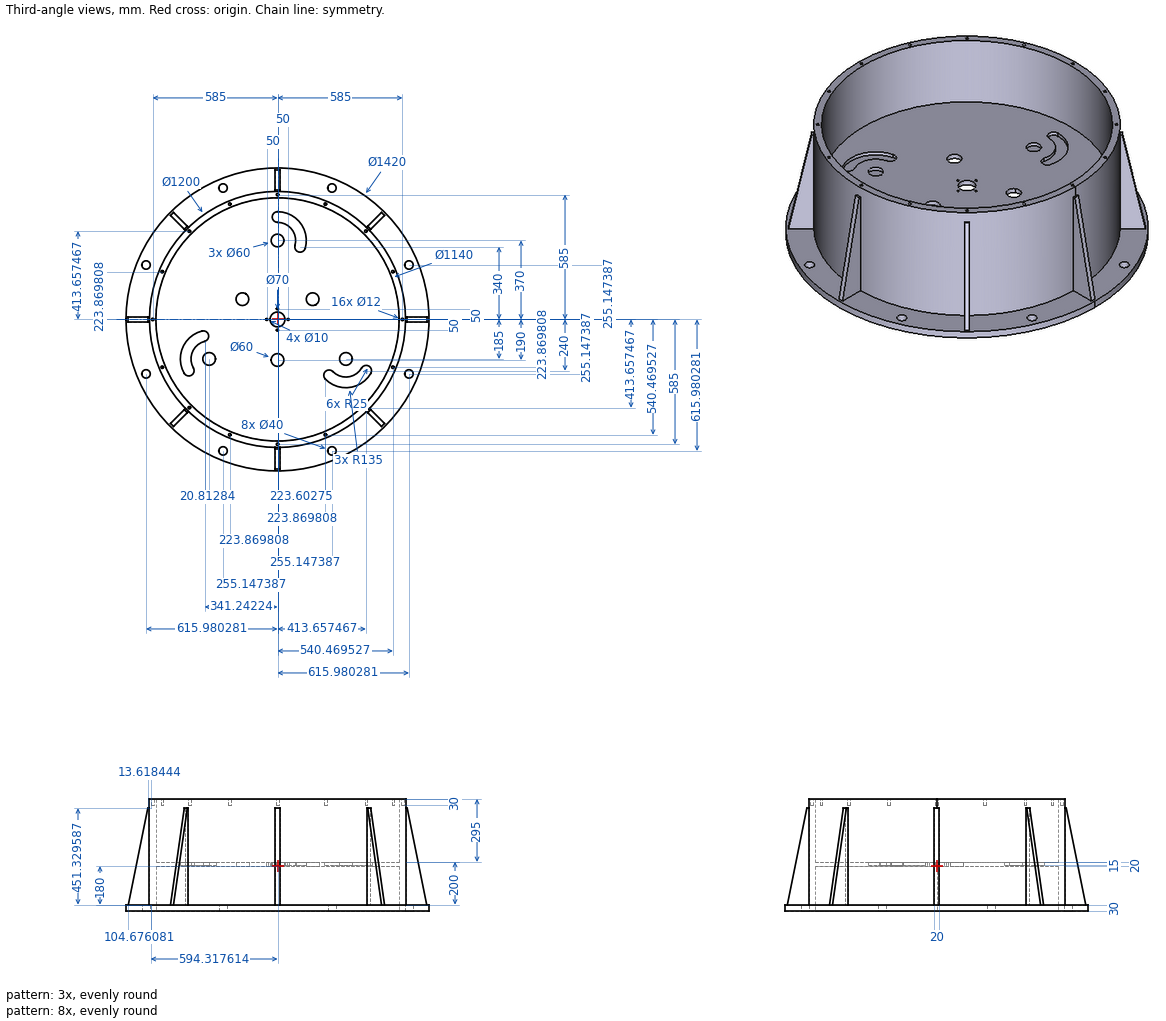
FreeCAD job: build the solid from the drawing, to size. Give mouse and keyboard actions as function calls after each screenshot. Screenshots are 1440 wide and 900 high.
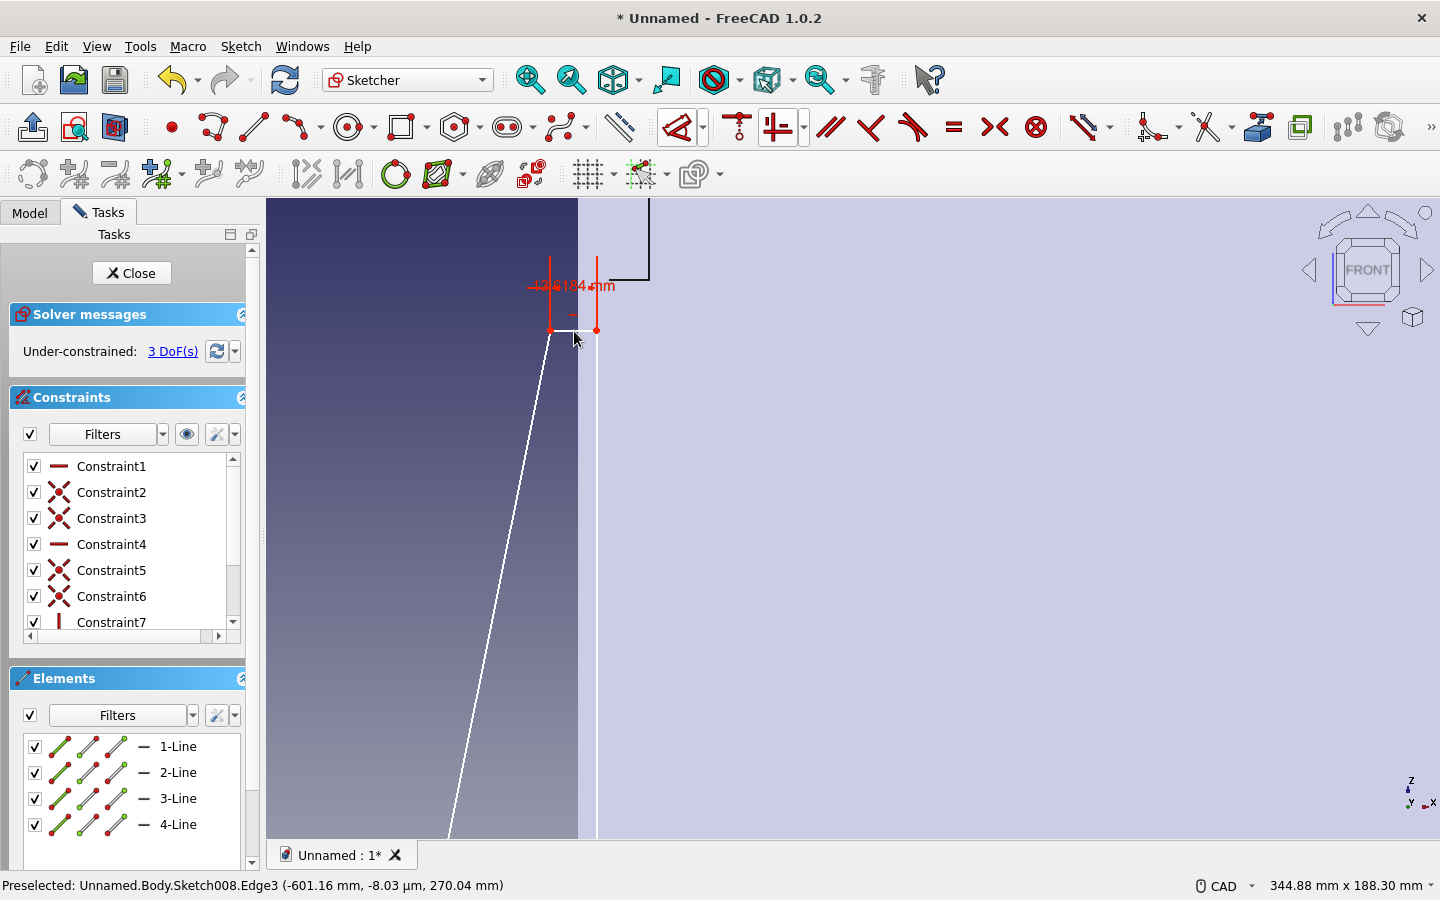
scroll(573, 330, down, 7)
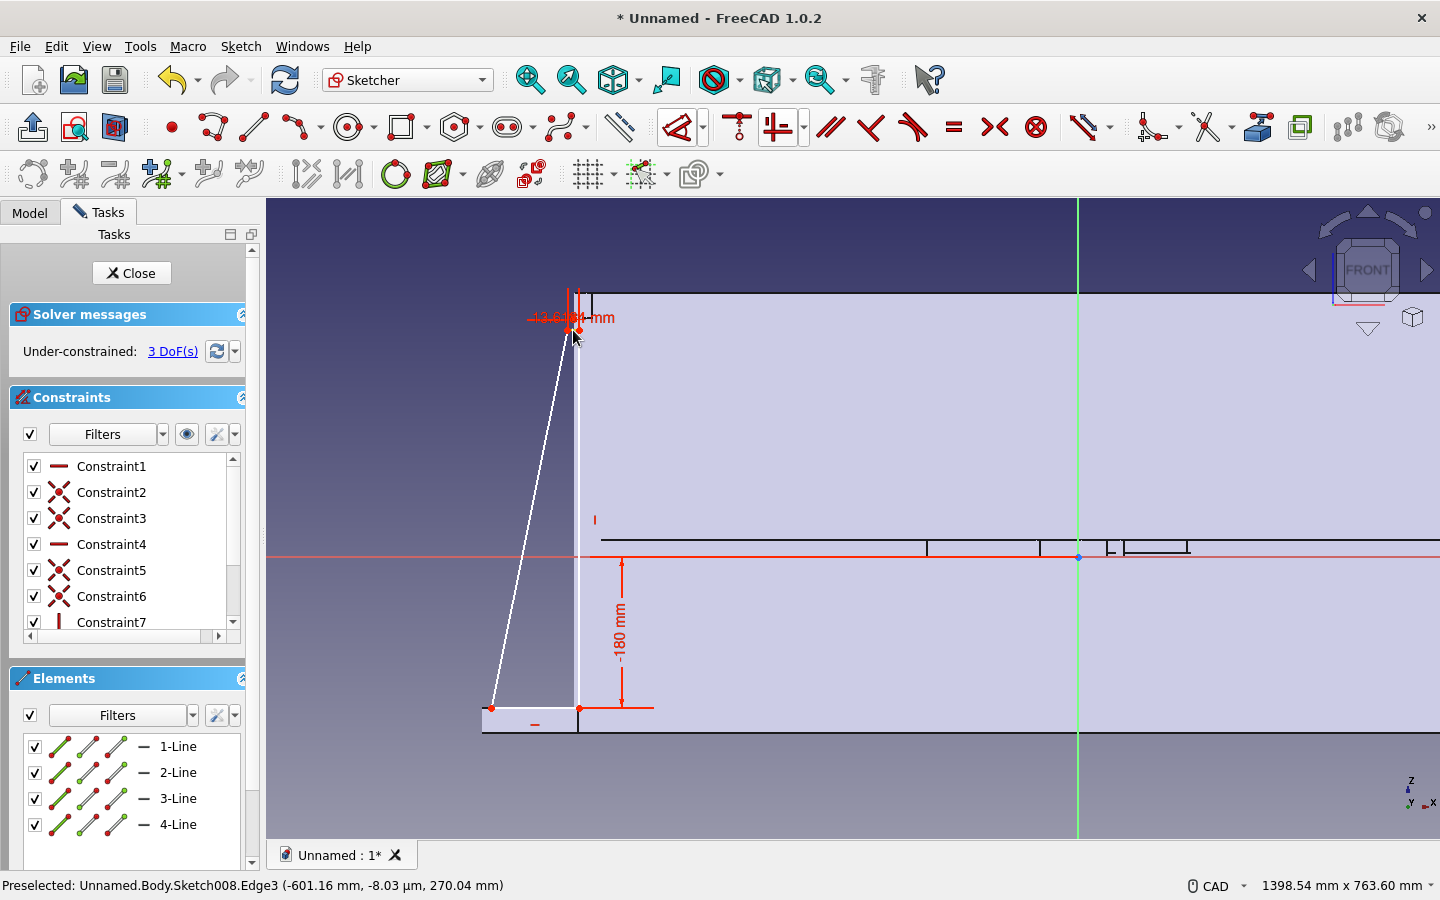
click(553, 708)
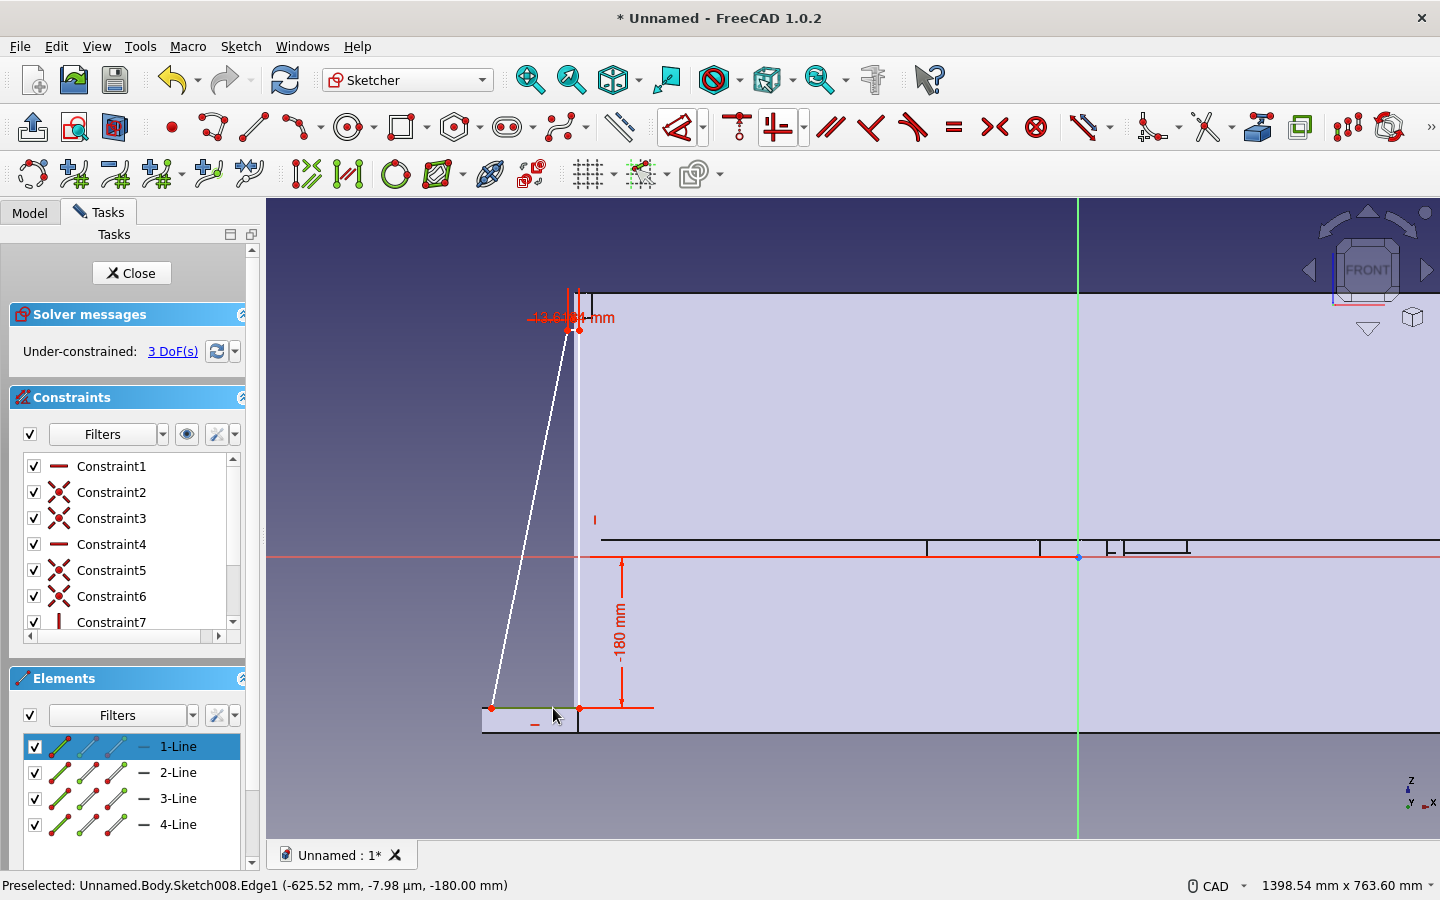
key(l)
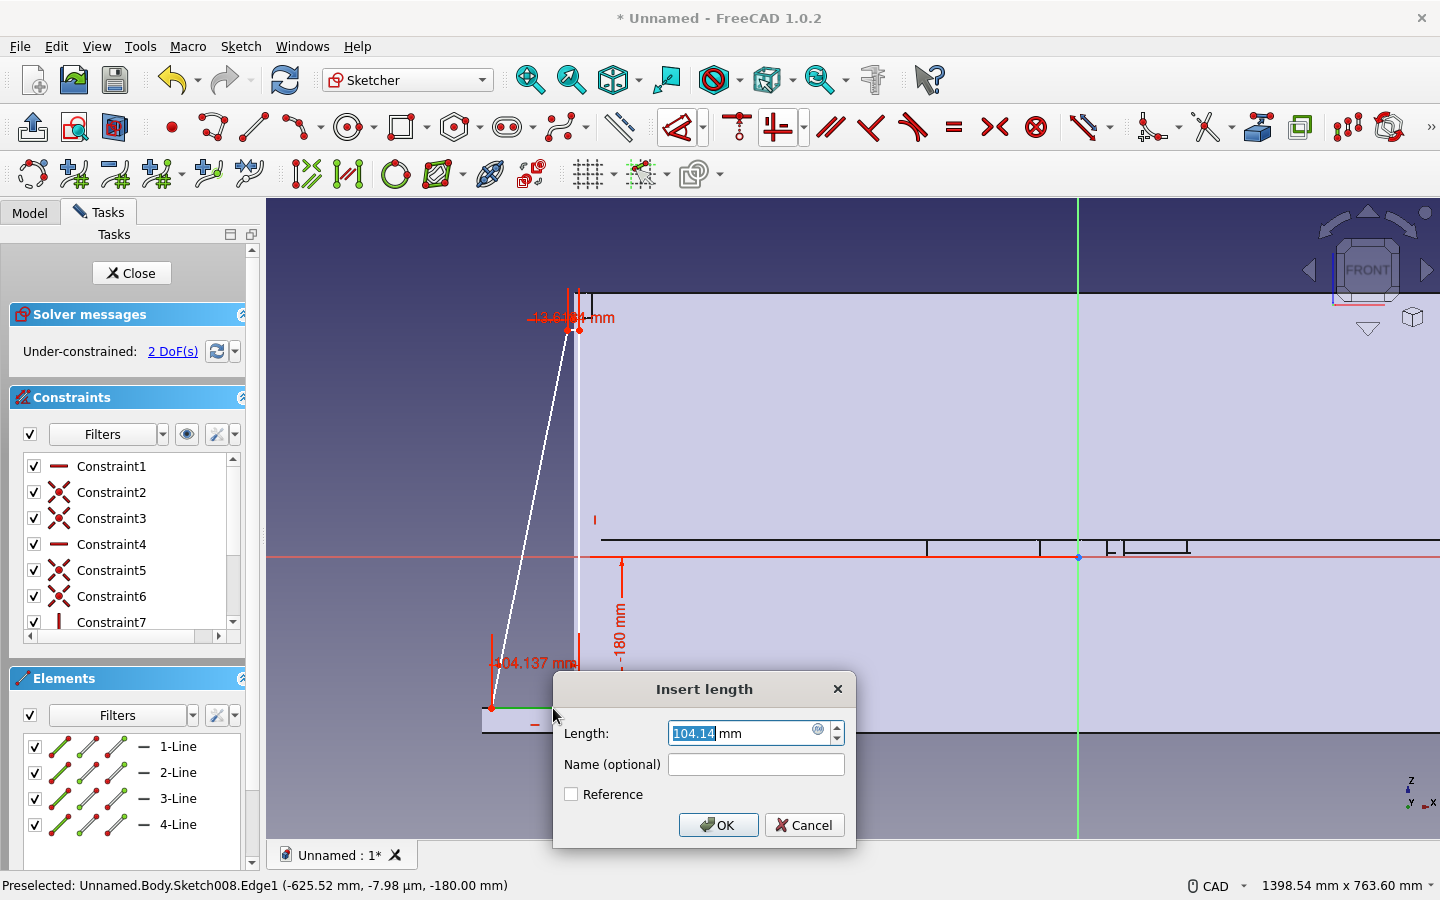
text(104.676081)
key(Return)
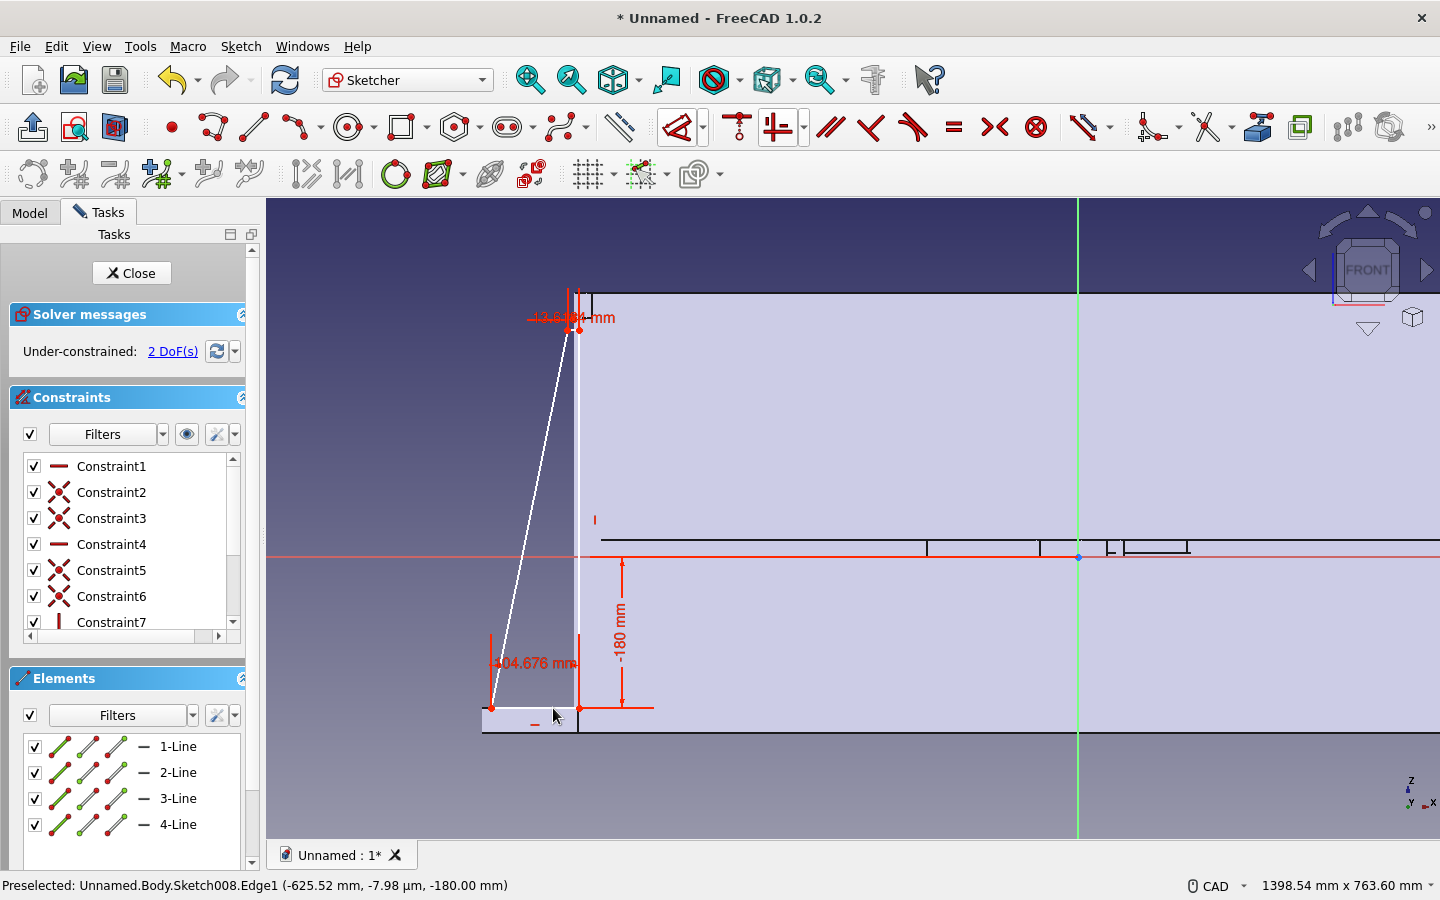
click(579, 444)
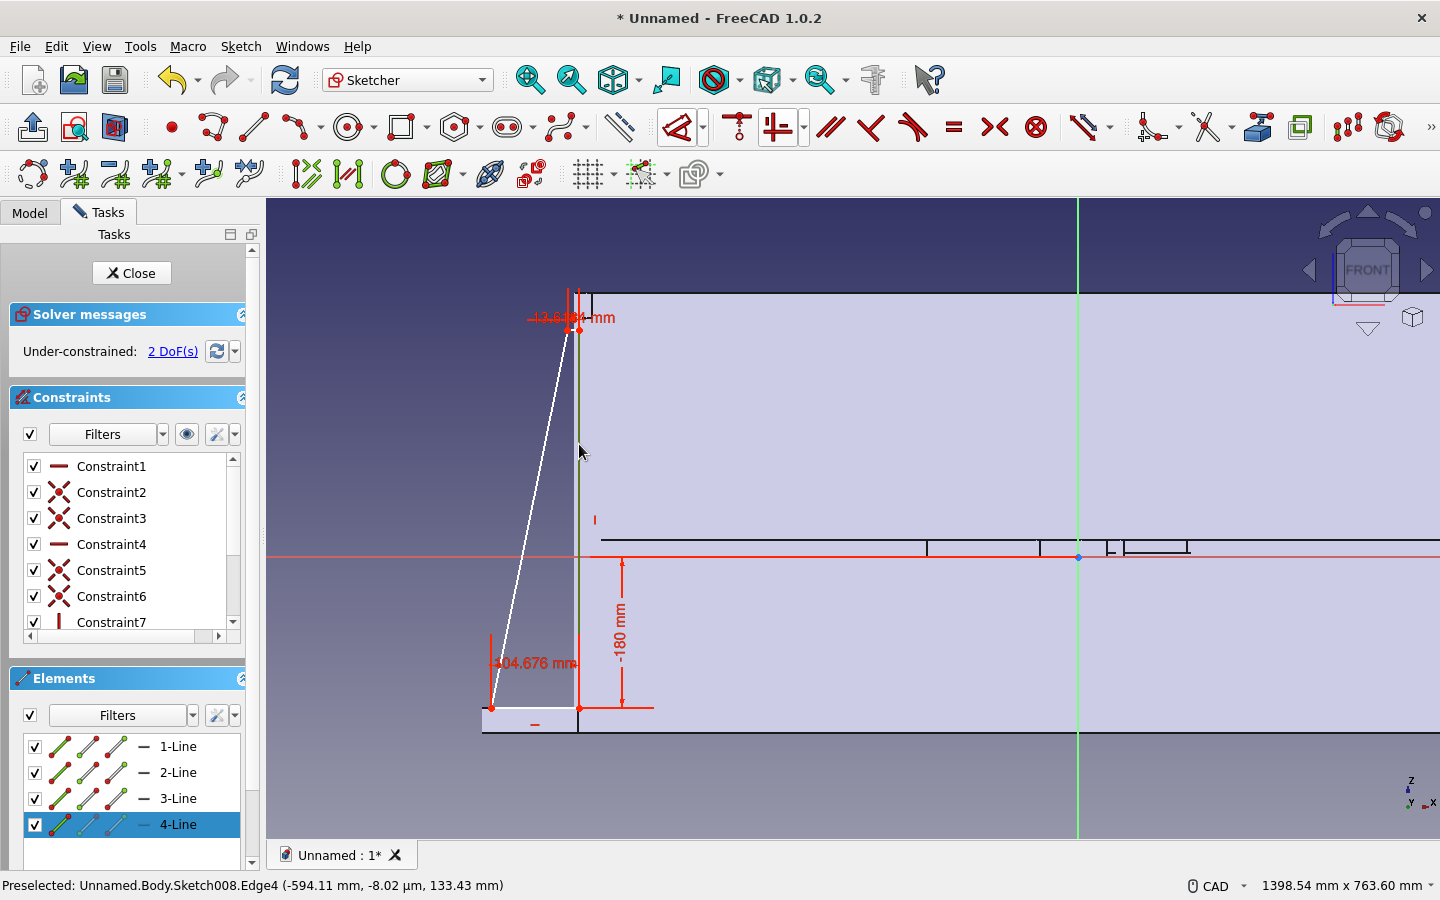
key(i)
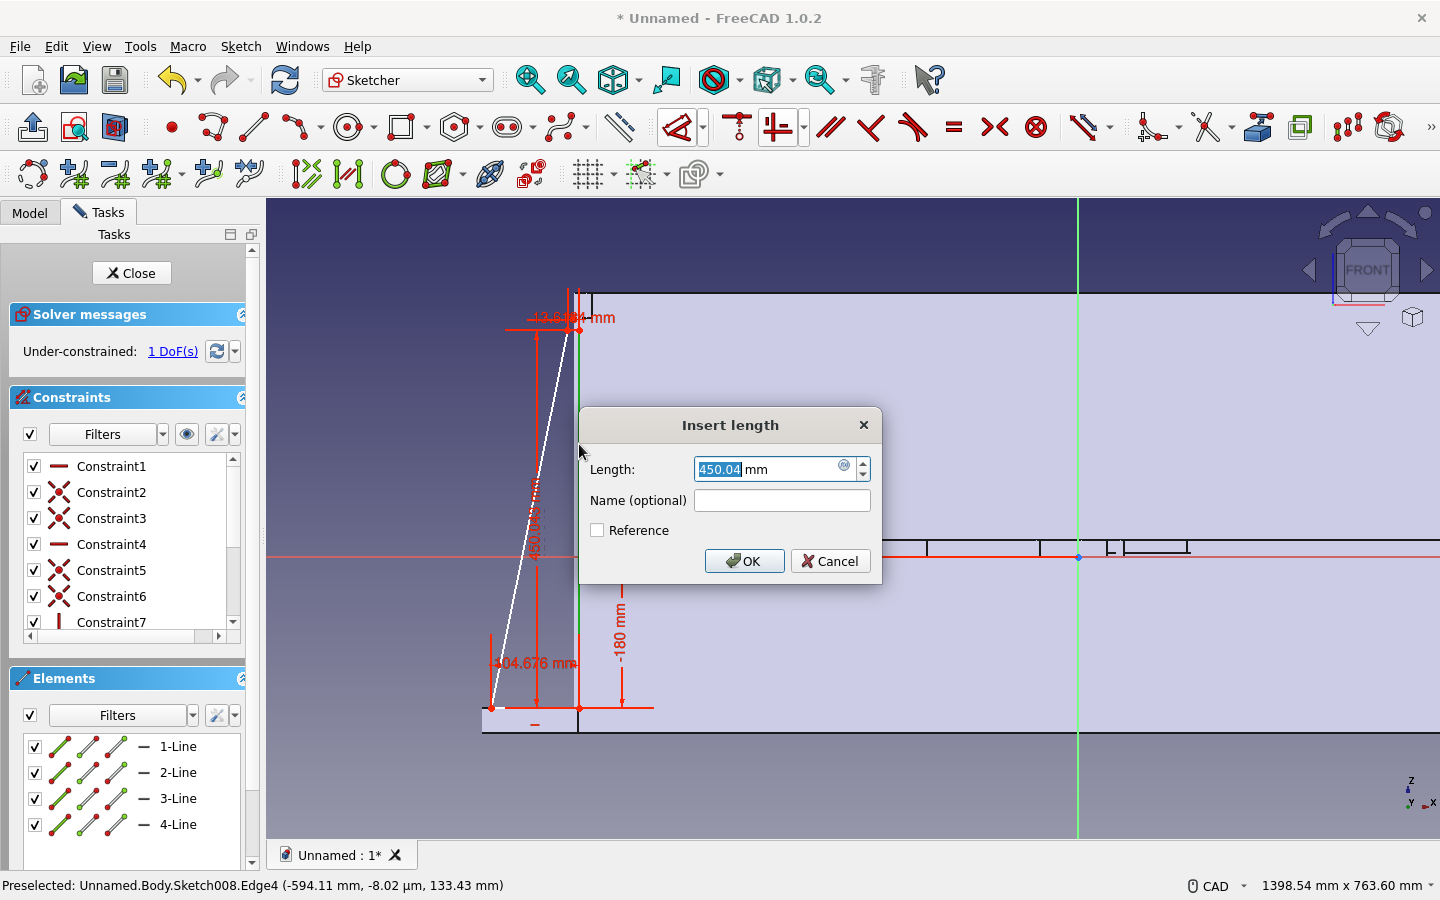
text(451.329587)
key(Return)